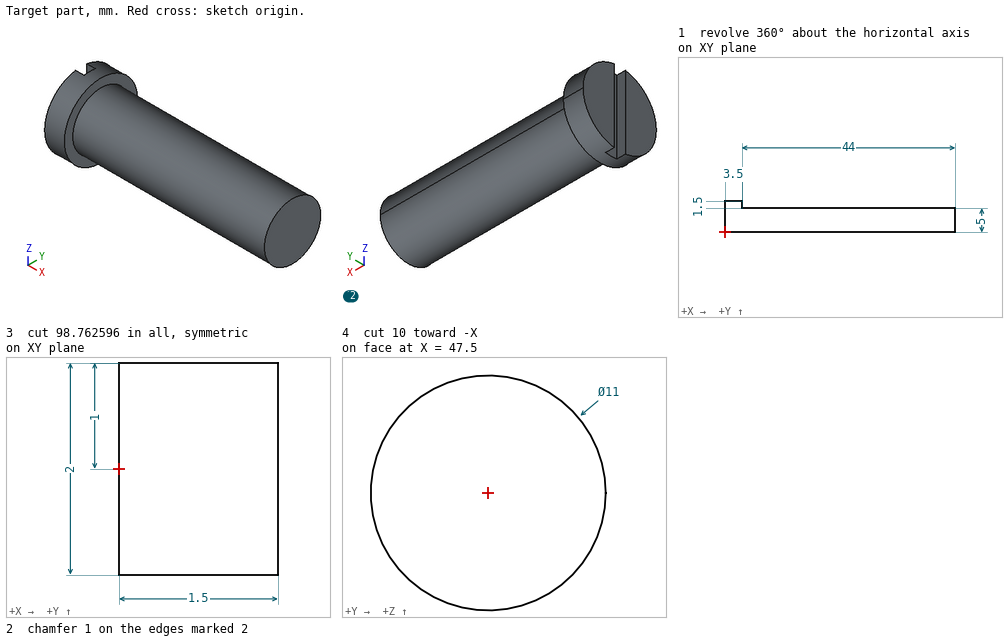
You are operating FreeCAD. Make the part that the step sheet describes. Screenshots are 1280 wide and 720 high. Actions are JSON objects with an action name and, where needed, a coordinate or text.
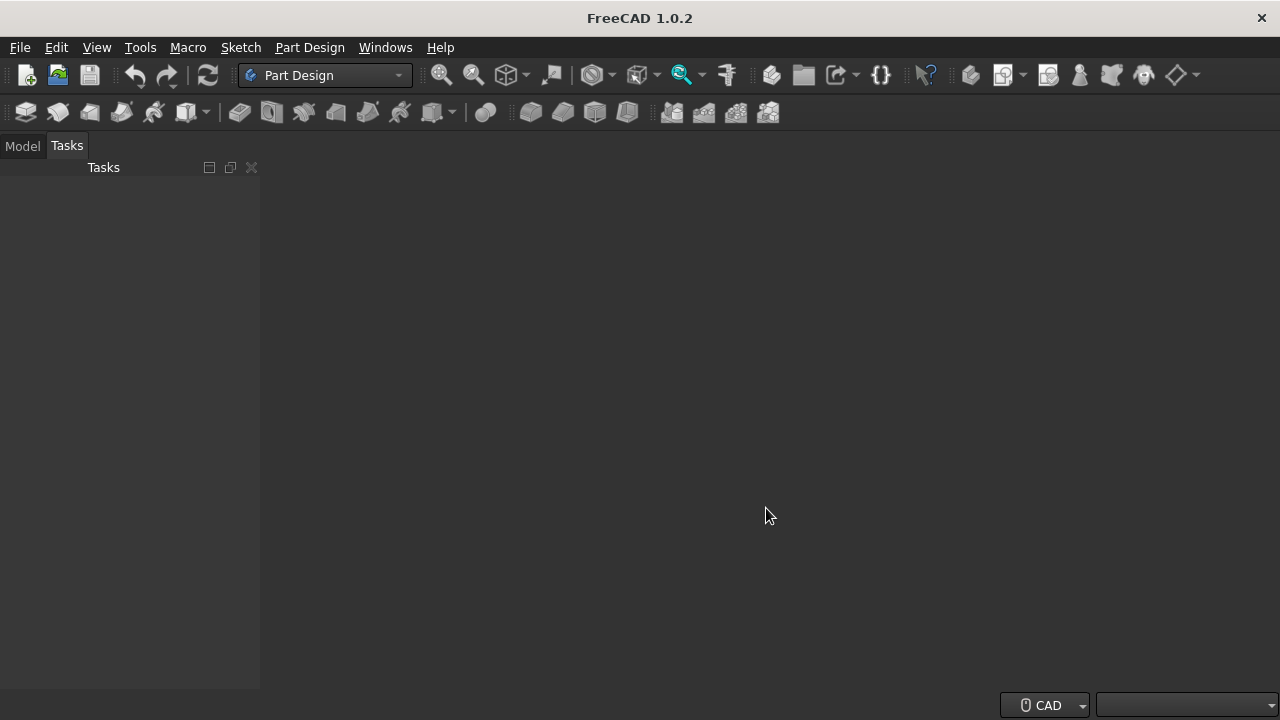
{"action": "left_click", "coordinate": [26, 76]}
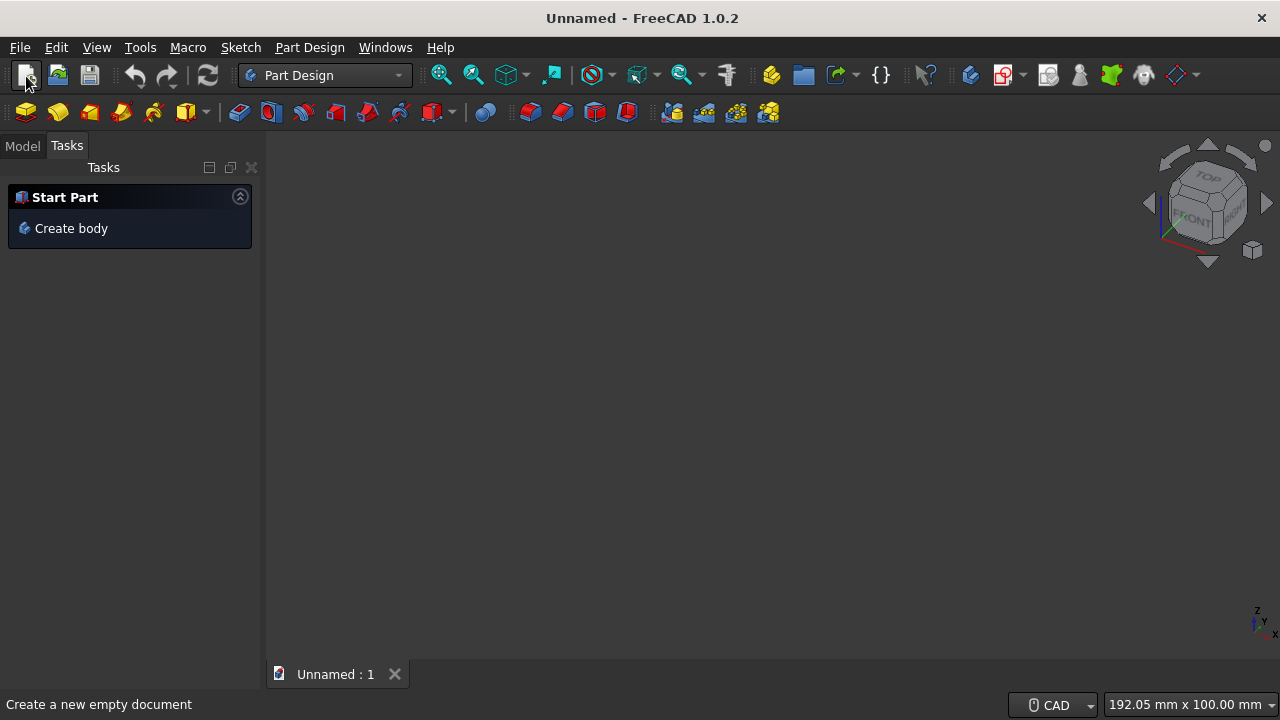
{"action": "left_click", "coordinate": [1004, 76]}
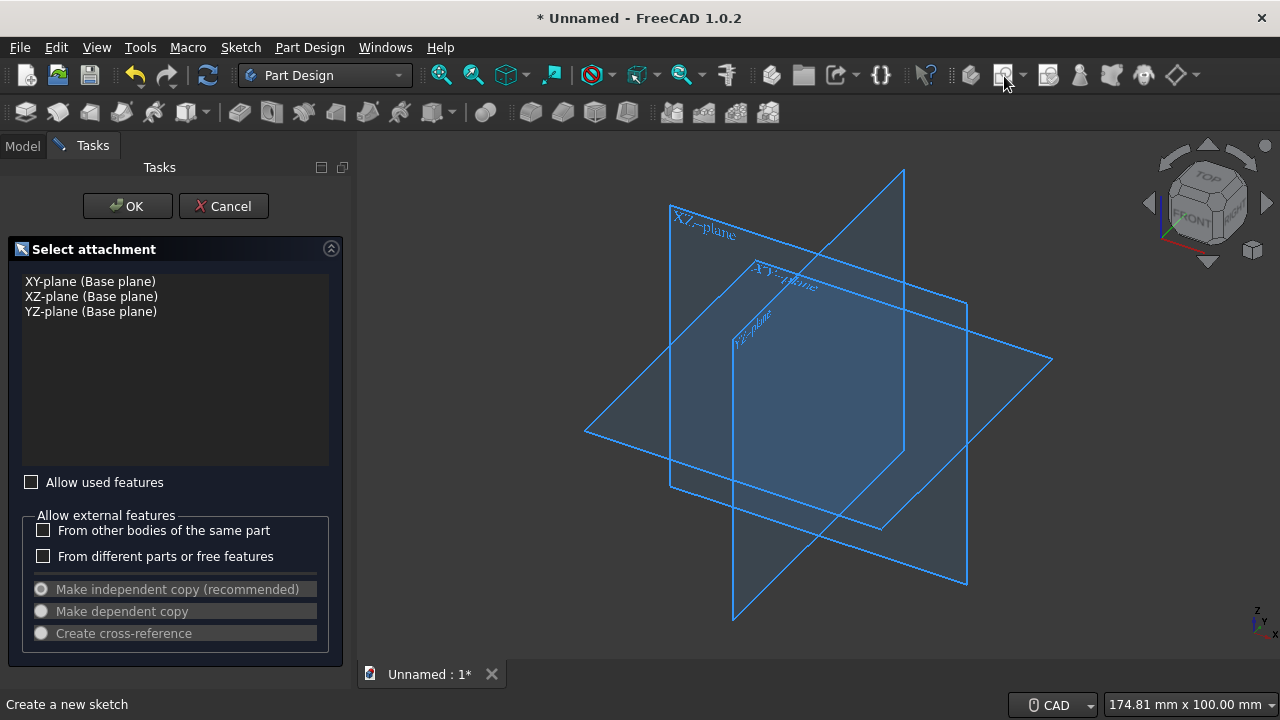
{"action": "left_click", "coordinate": [82, 282]}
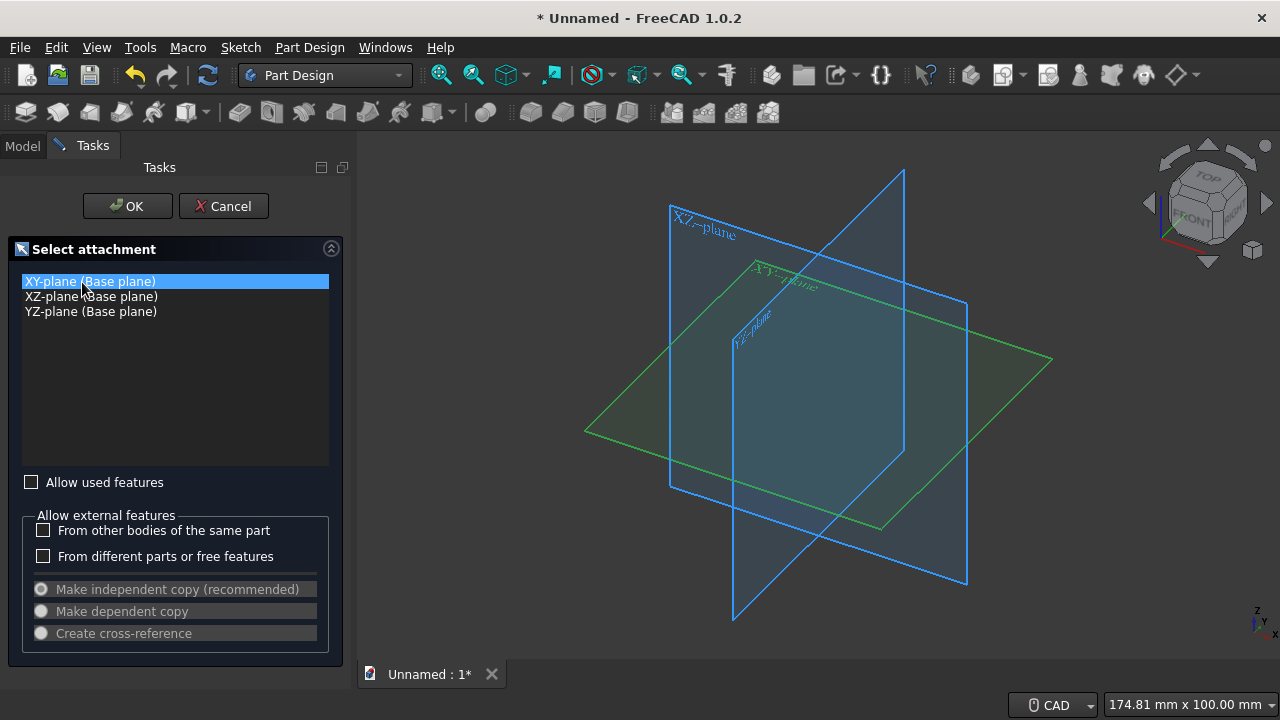
{"action": "left_click", "coordinate": [128, 206]}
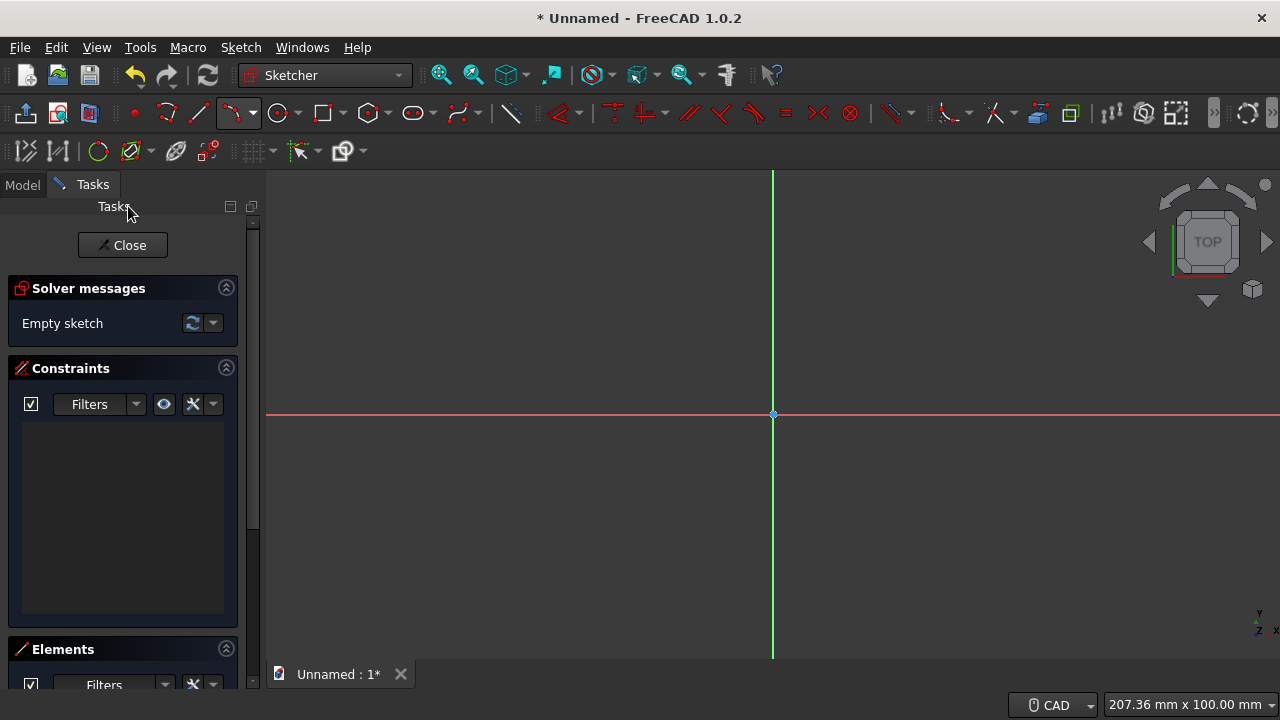
{"action": "scroll", "coordinate": [997, 389], "scroll_direction": "up", "scroll_amount": 5}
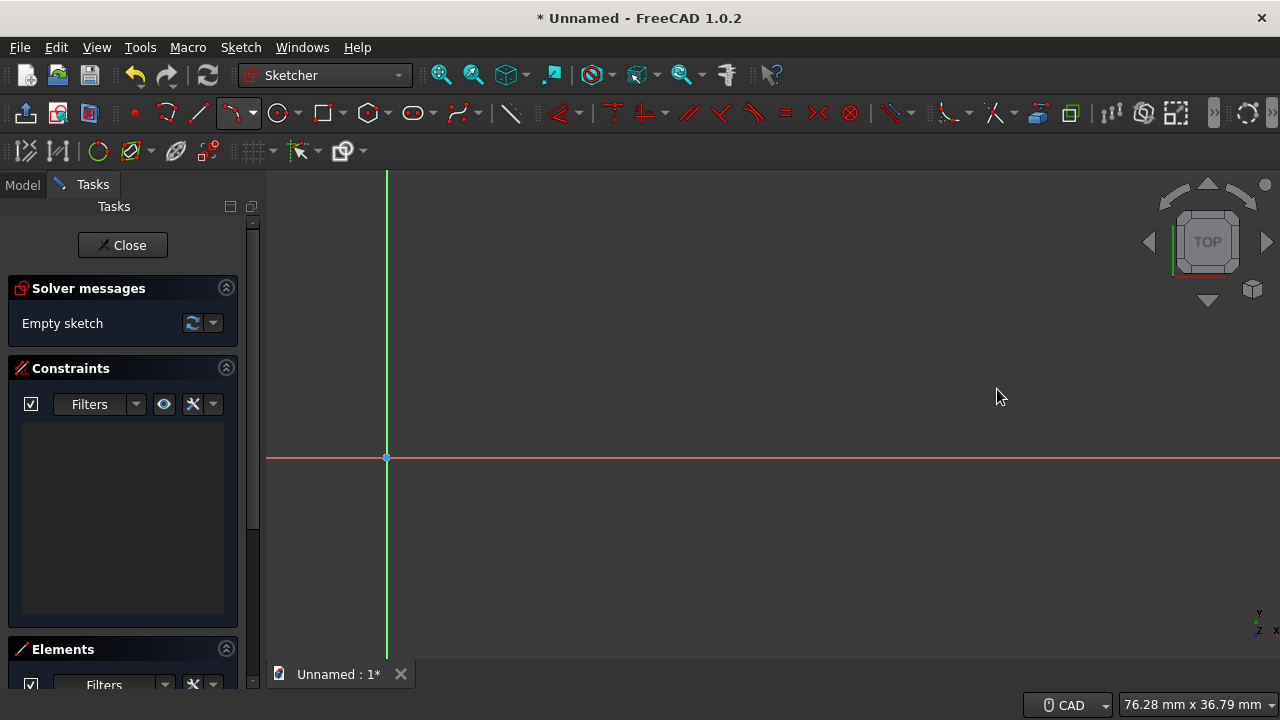
{"action": "key", "text": "g m"}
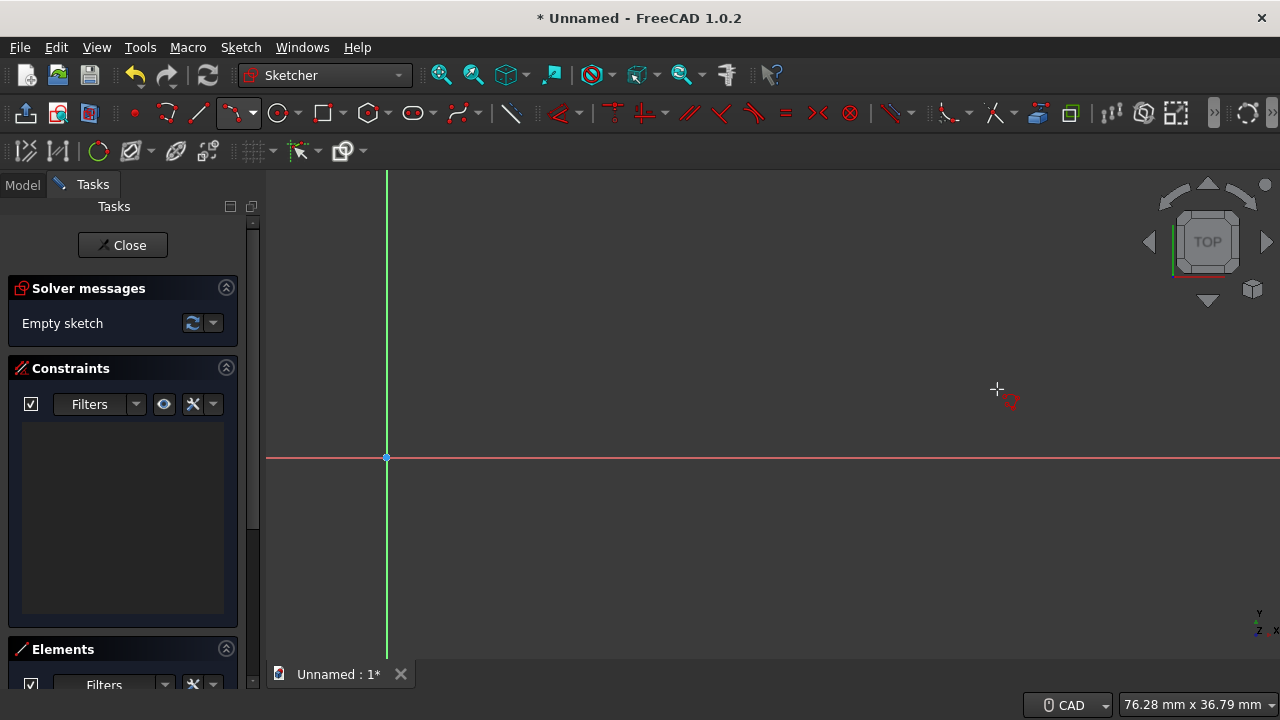
{"action": "left_click", "coordinate": [387, 458]}
{"action": "left_click", "coordinate": [1018, 449]}
{"action": "left_click", "coordinate": [1018, 391]}
{"action": "left_click", "coordinate": [433, 391]}
{"action": "left_click", "coordinate": [433, 371]}
{"action": "left_click", "coordinate": [396, 371]}
{"action": "left_click", "coordinate": [387, 458]}
{"action": "key", "text": "Escape"}
{"action": "key", "text": "Escape"}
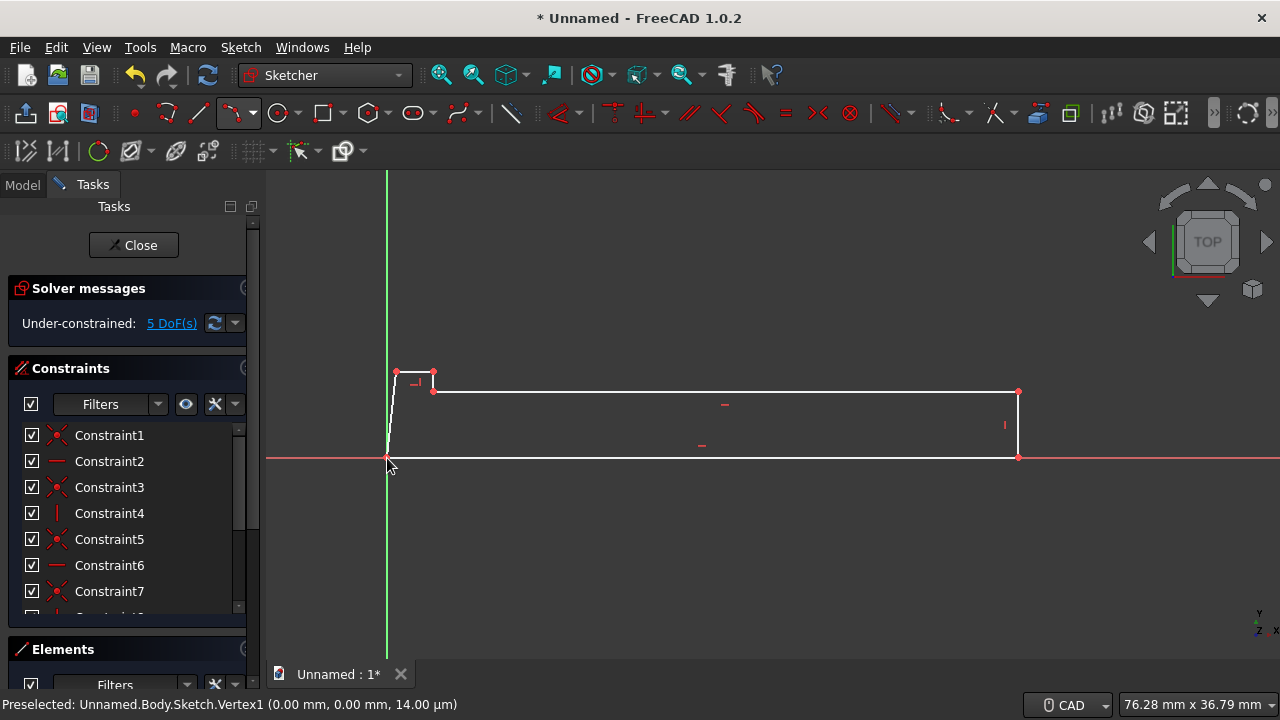
{"action": "left_click", "coordinate": [390, 432]}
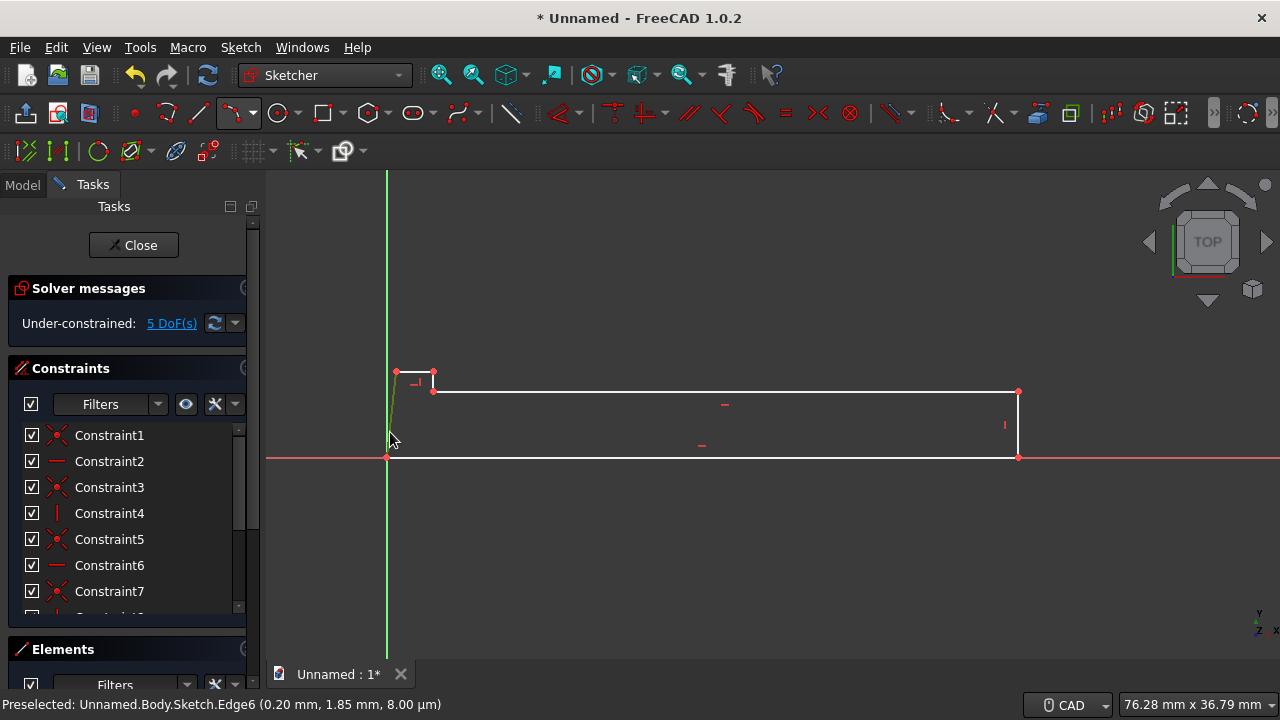
{"action": "key", "text": "v"}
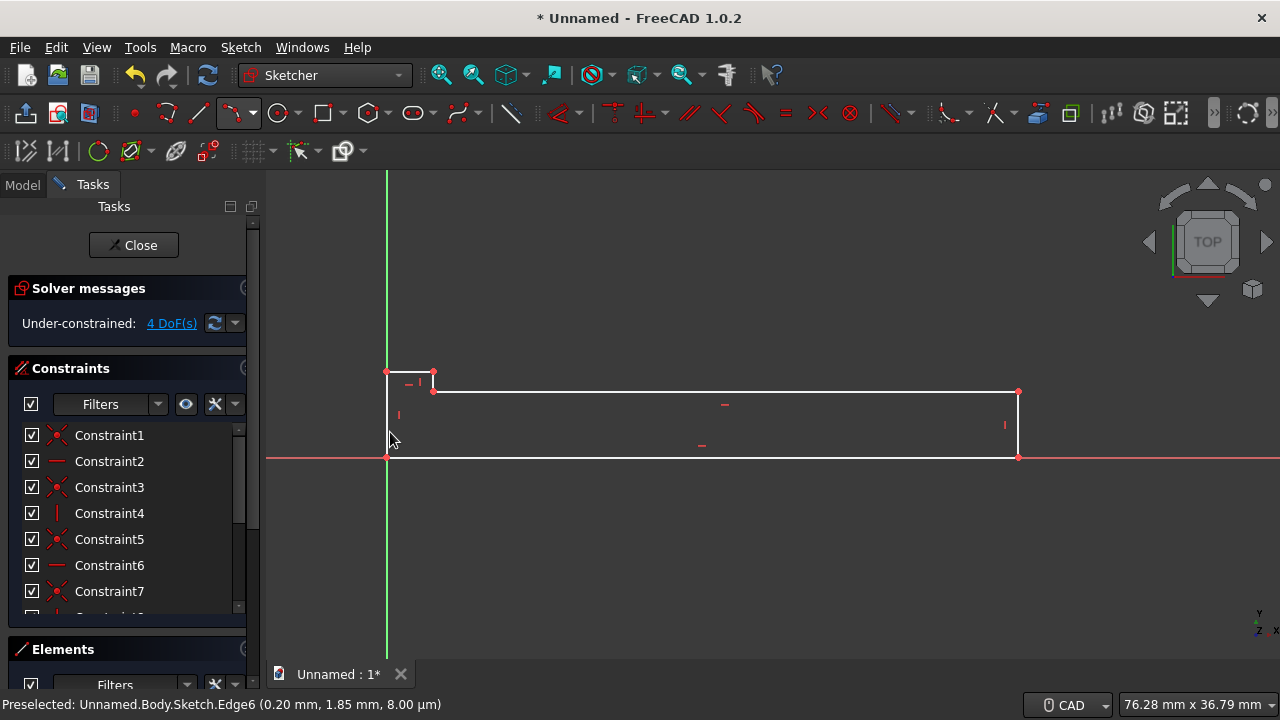
{"action": "left_click", "coordinate": [558, 114]}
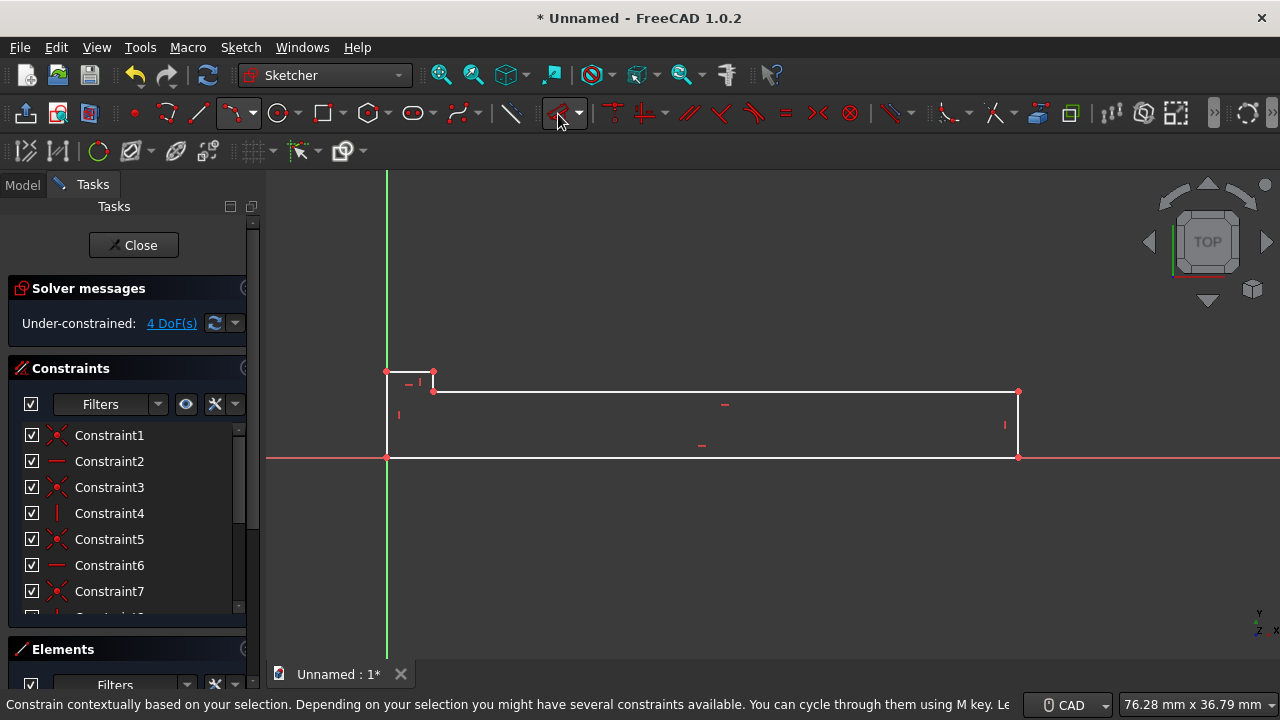
{"action": "left_click", "coordinate": [1018, 438]}
{"action": "left_click", "coordinate": [1052, 425]}